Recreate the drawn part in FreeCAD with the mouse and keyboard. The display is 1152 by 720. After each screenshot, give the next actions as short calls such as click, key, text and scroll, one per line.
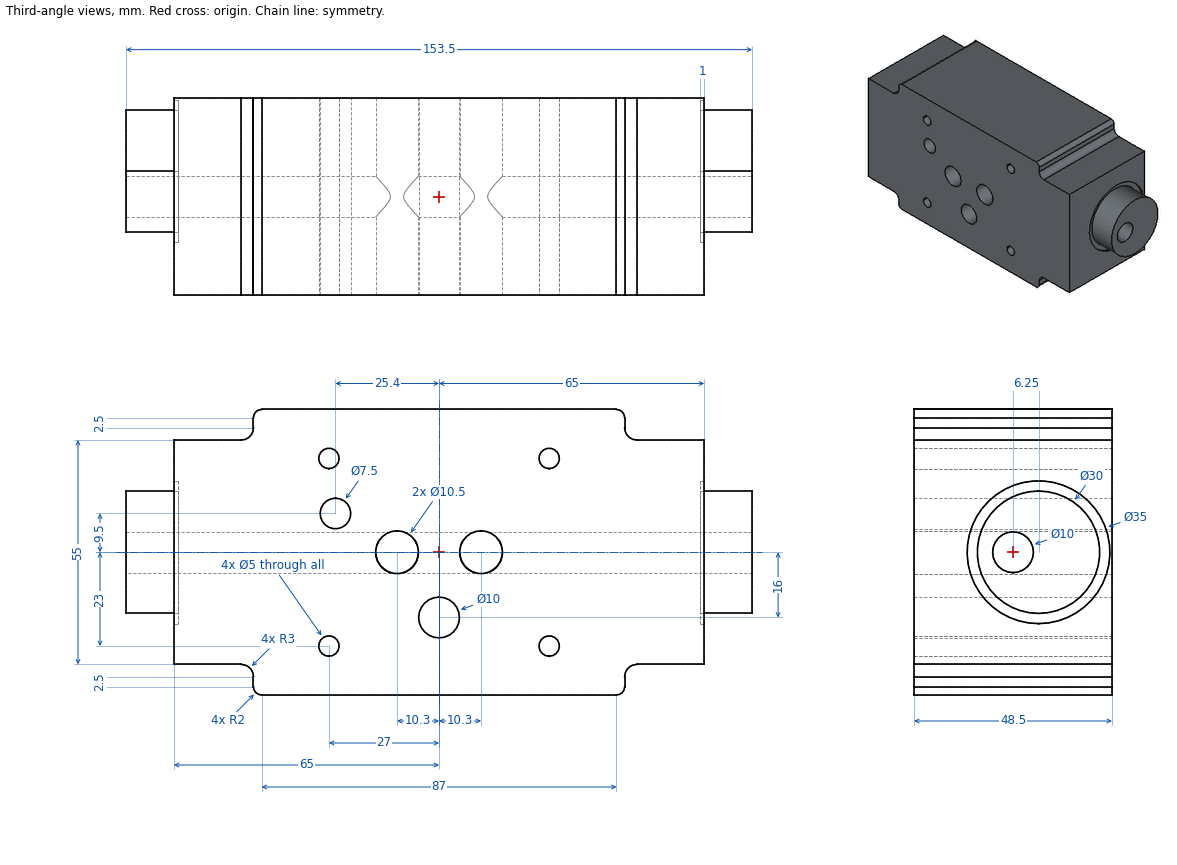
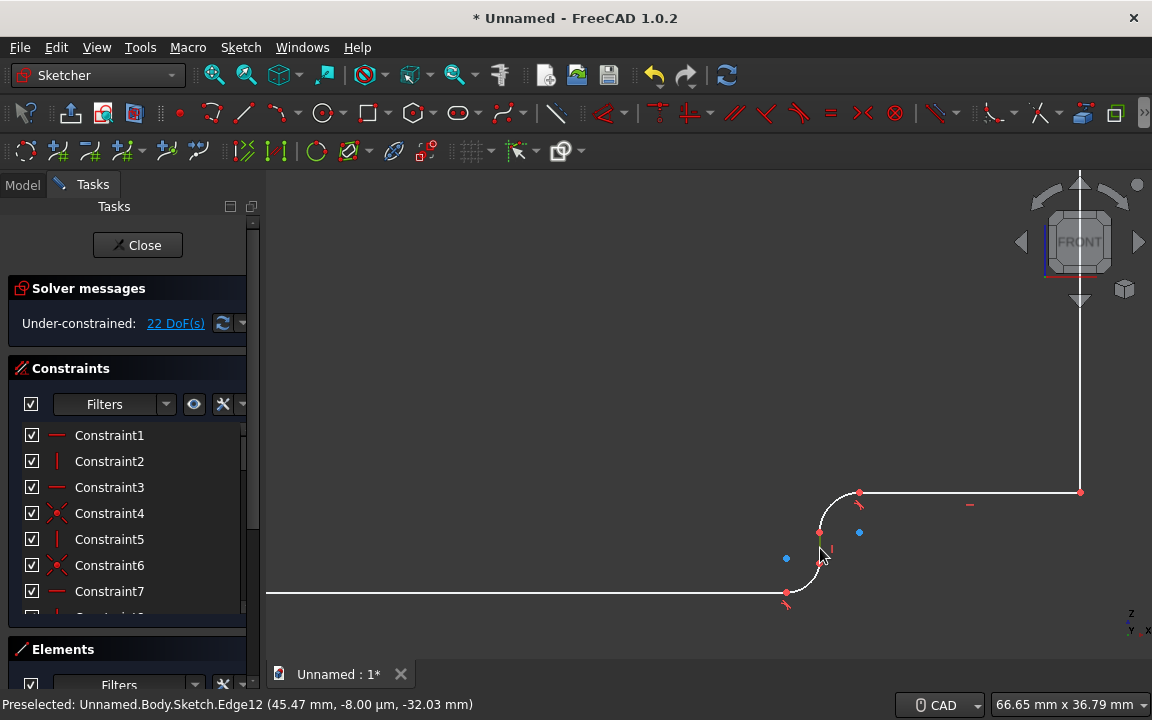
click(842, 497)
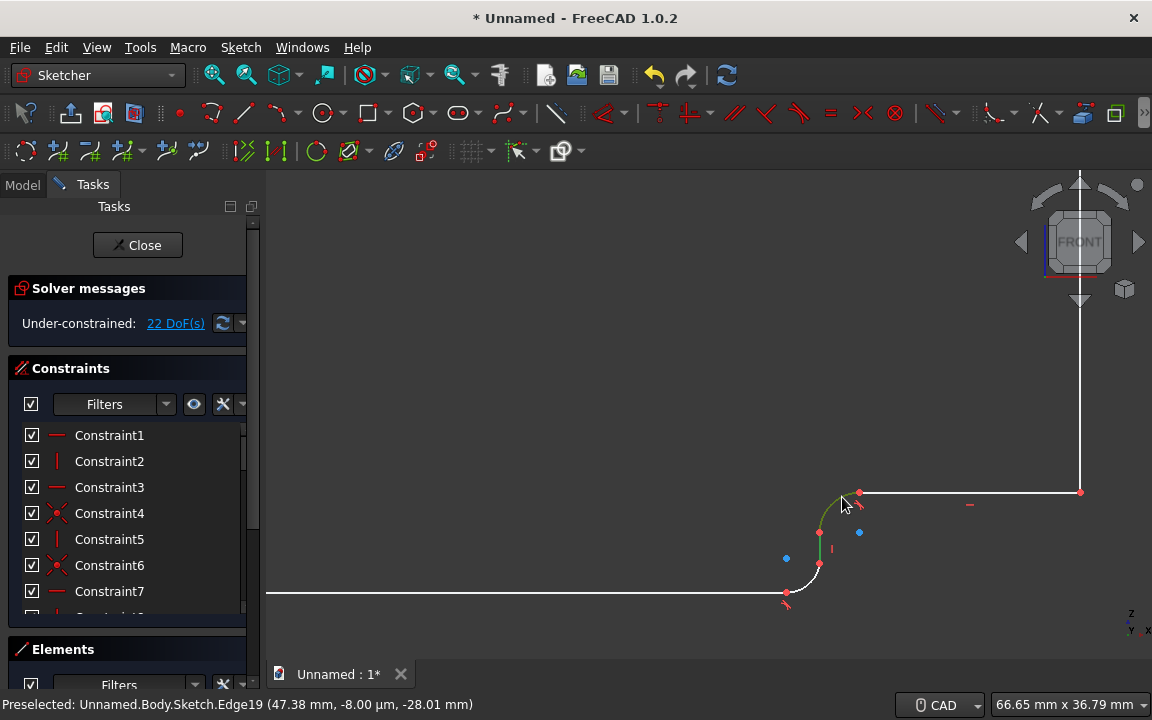
click(800, 114)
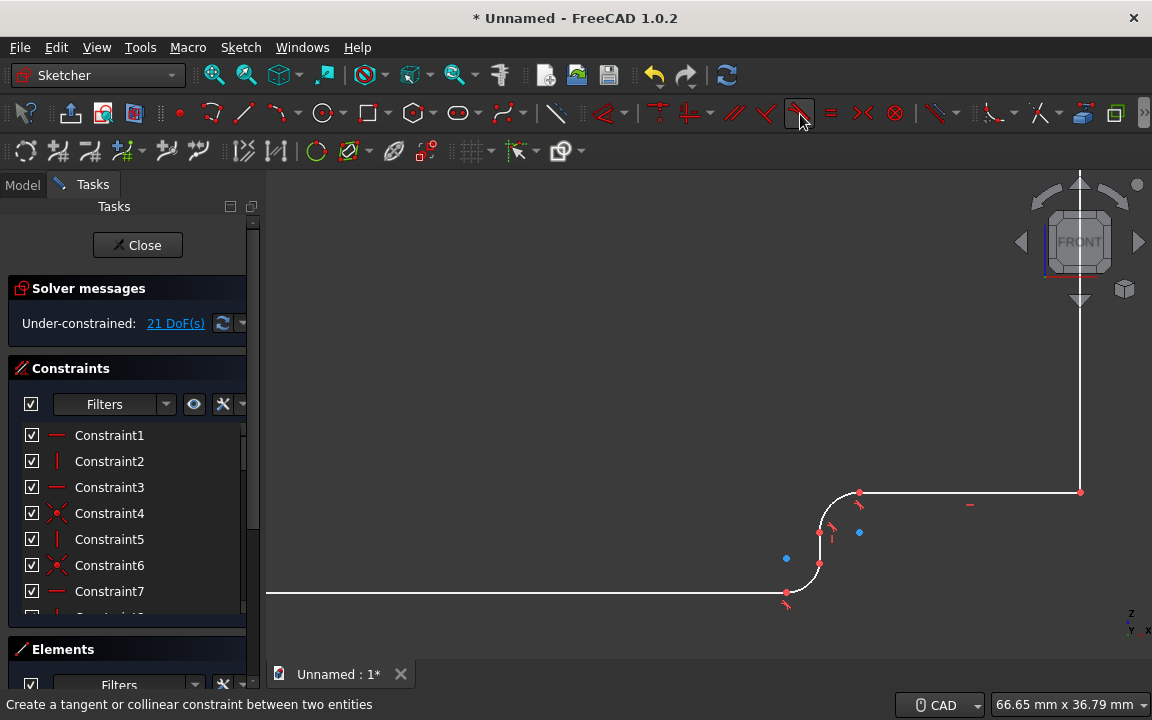
scroll(820, 542, up, 2)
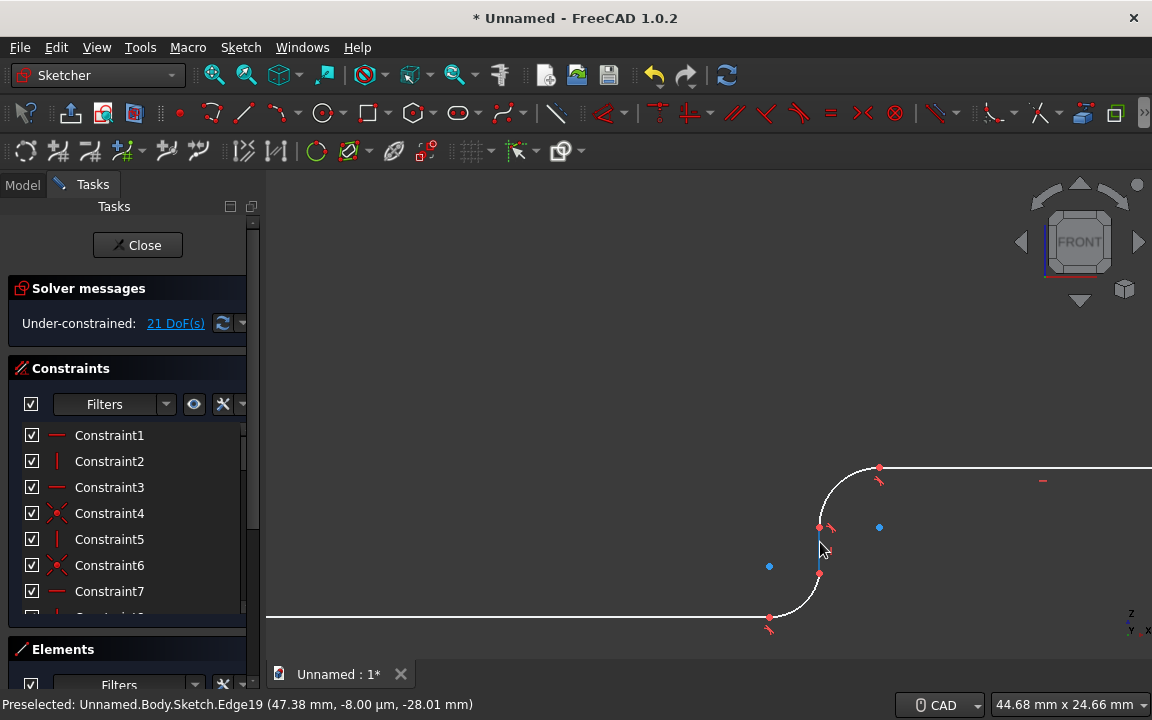
click(819, 542)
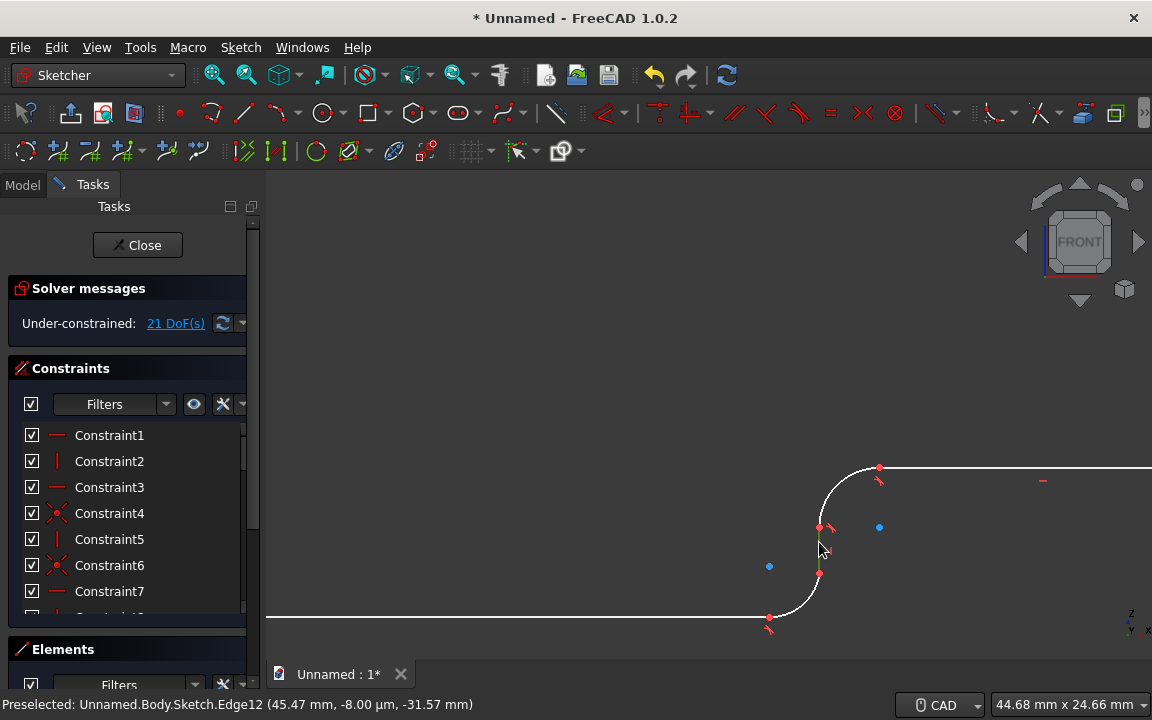
click(790, 613)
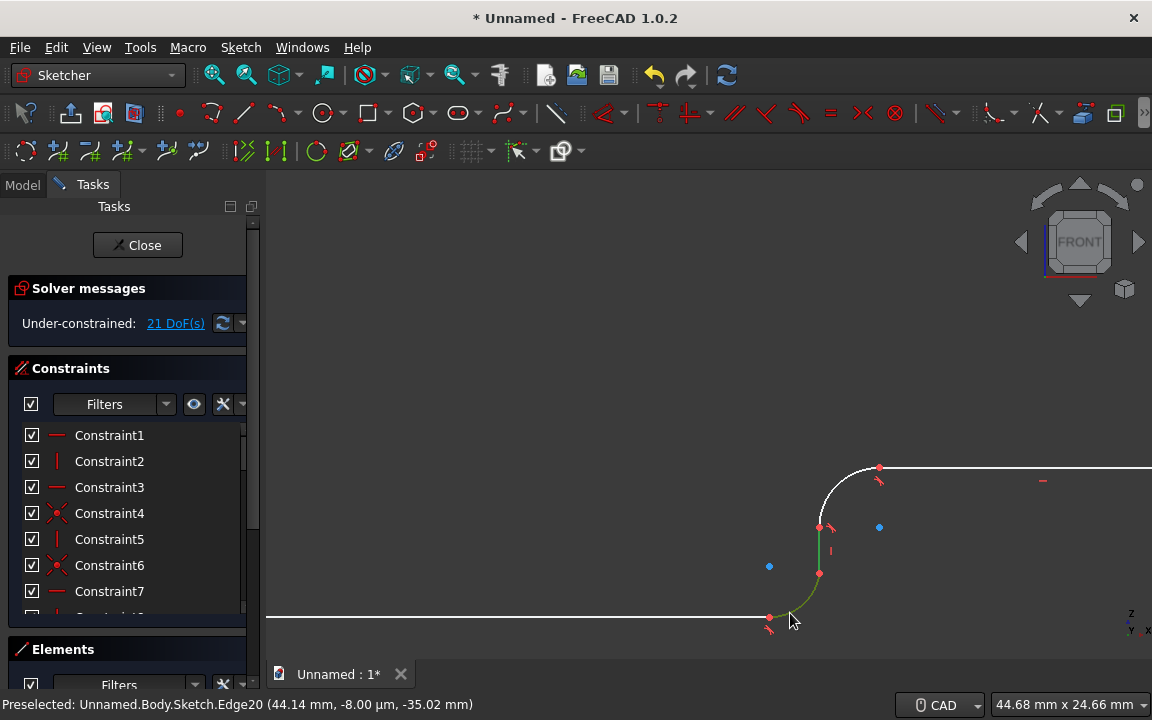
click(800, 114)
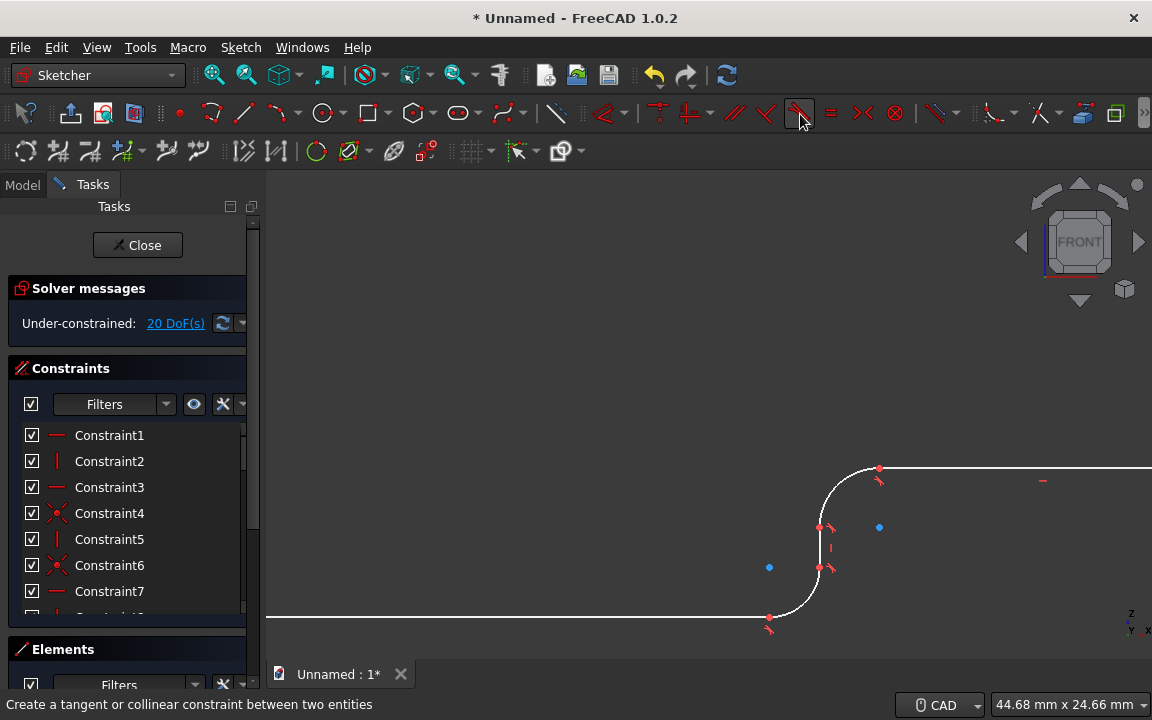
scroll(823, 540, down, 8)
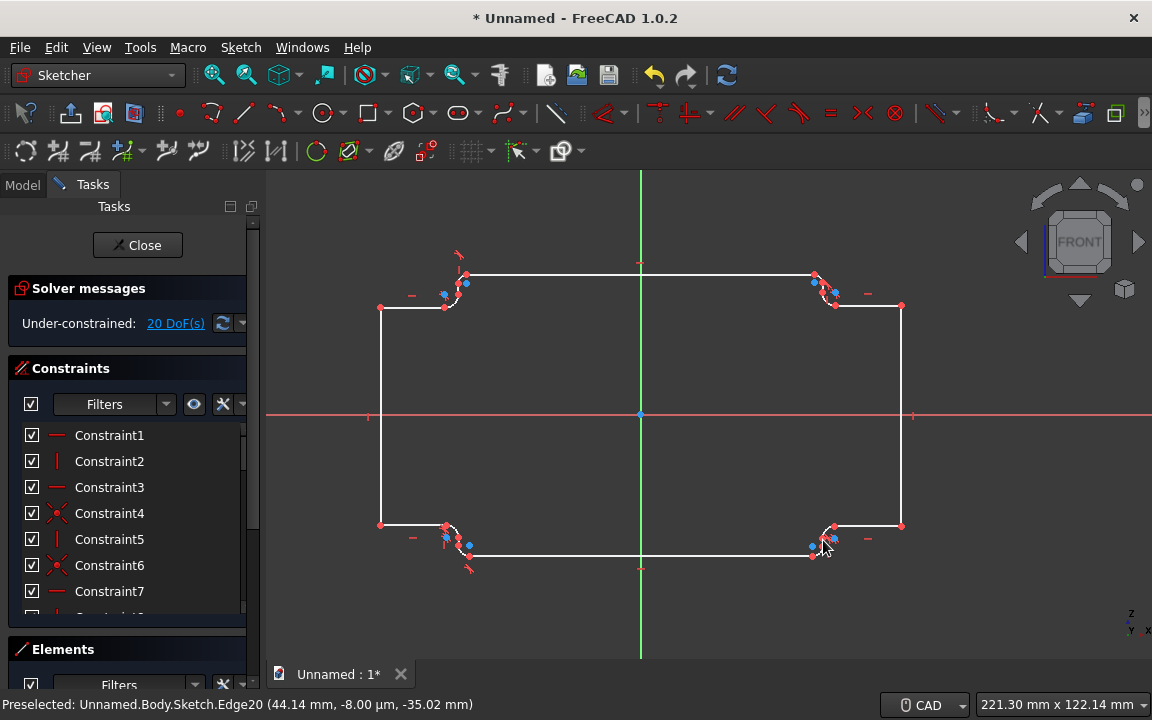
scroll(457, 532, up, 5)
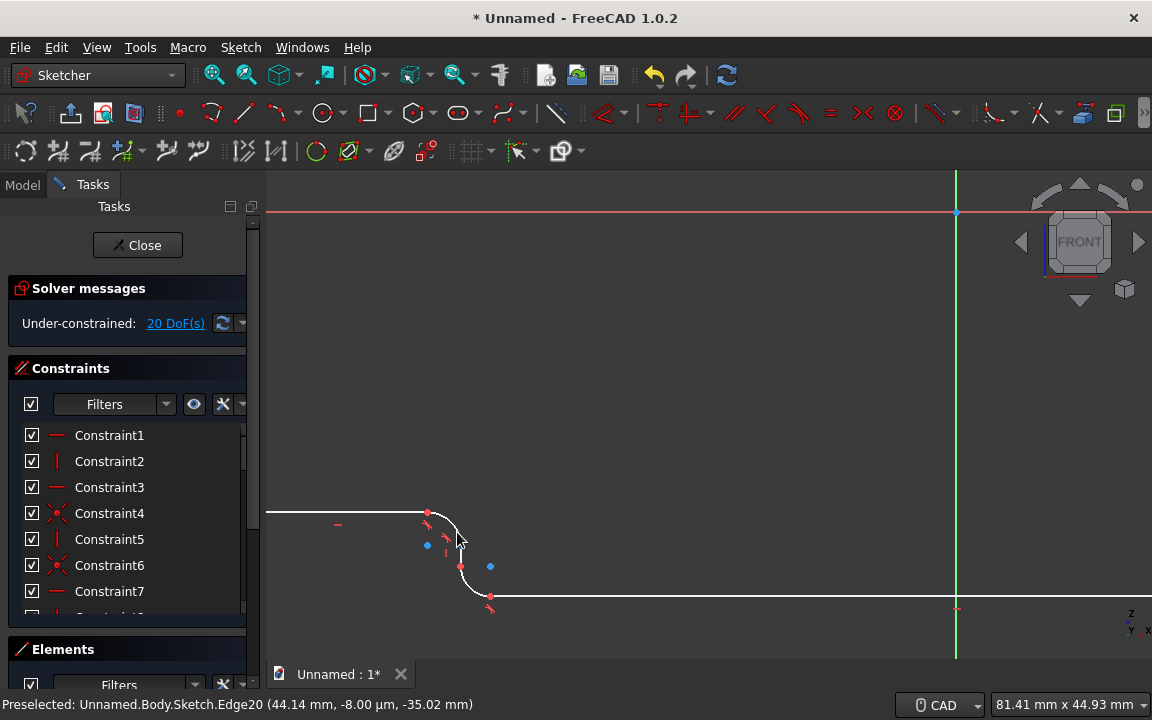
click(457, 531)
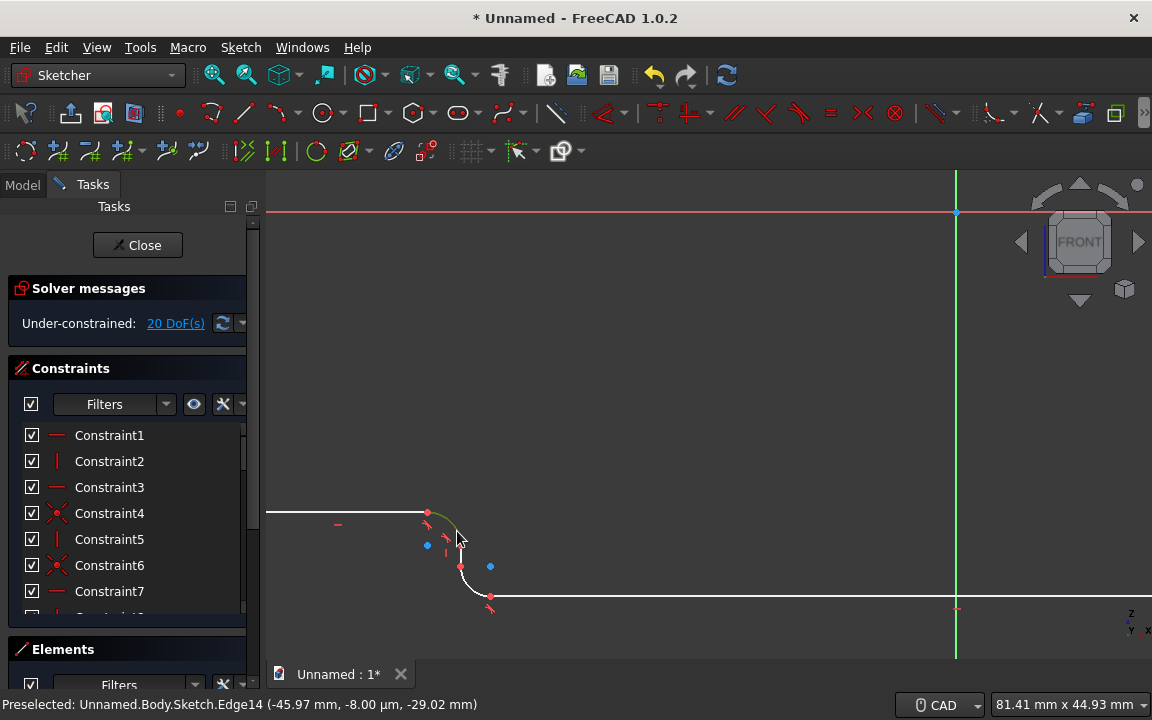
scroll(457, 532, down, 5)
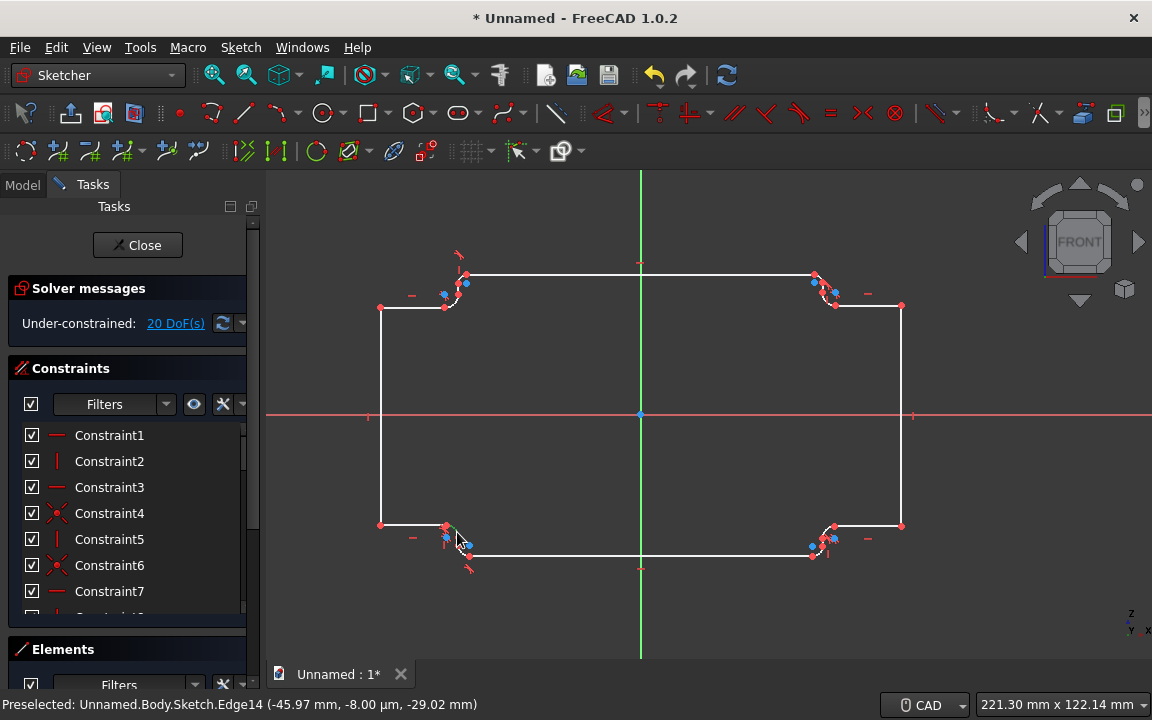
scroll(451, 306, up, 4)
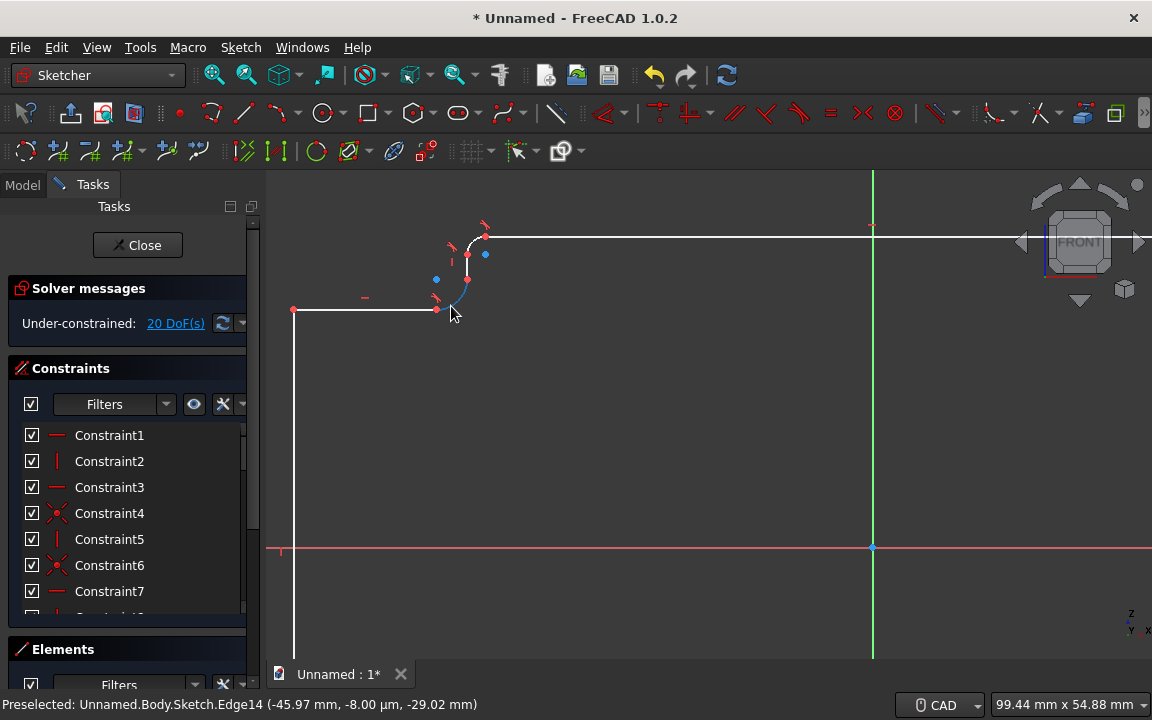
click(450, 307)